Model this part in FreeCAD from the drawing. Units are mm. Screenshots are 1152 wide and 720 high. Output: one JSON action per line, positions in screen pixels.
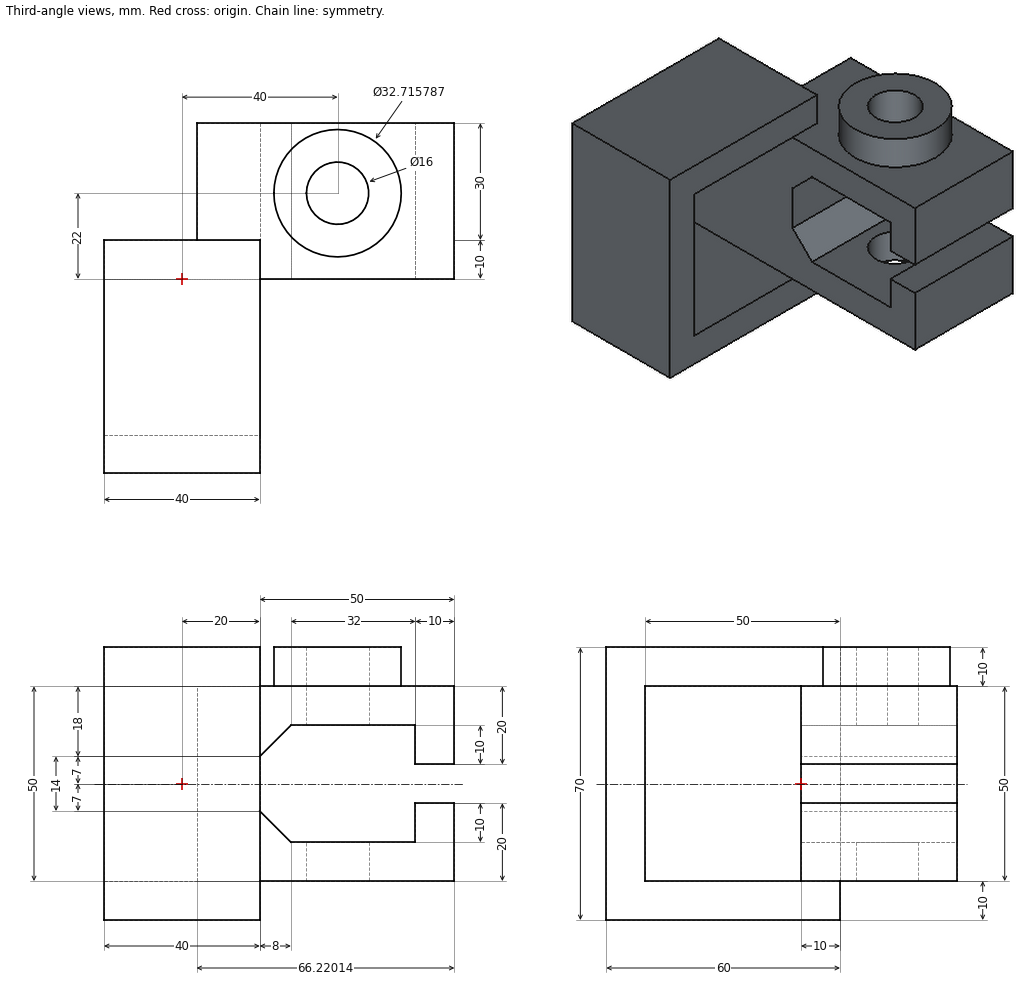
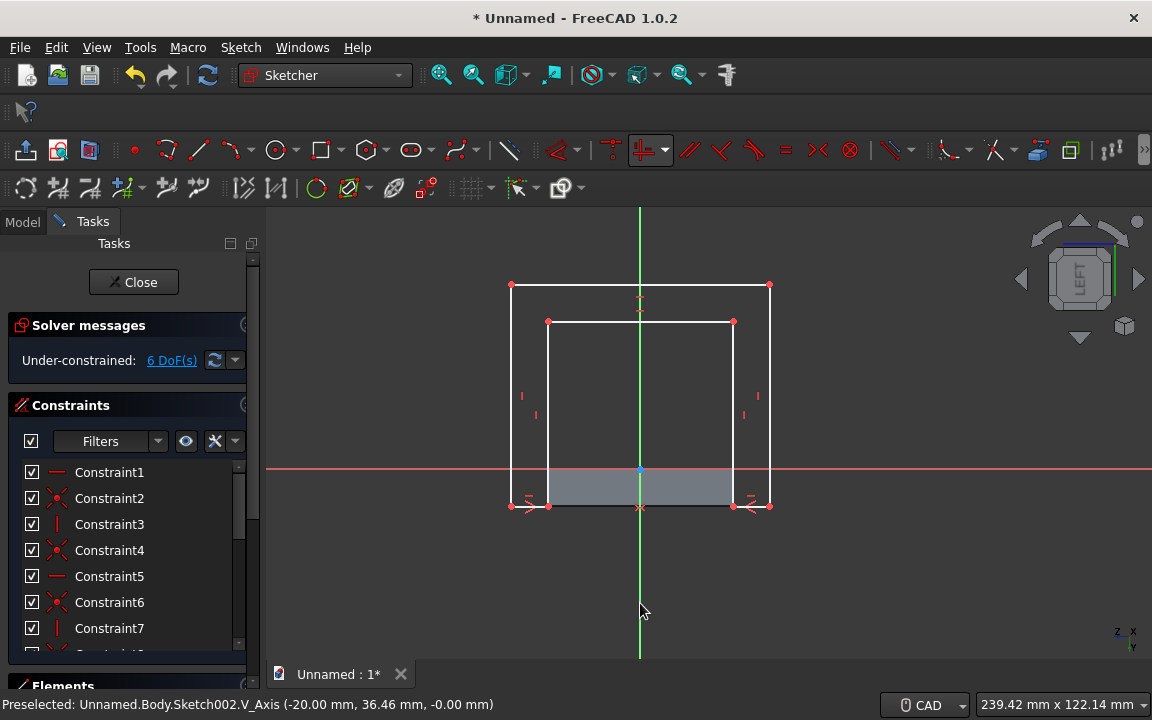
{"action": "key", "text": "d"}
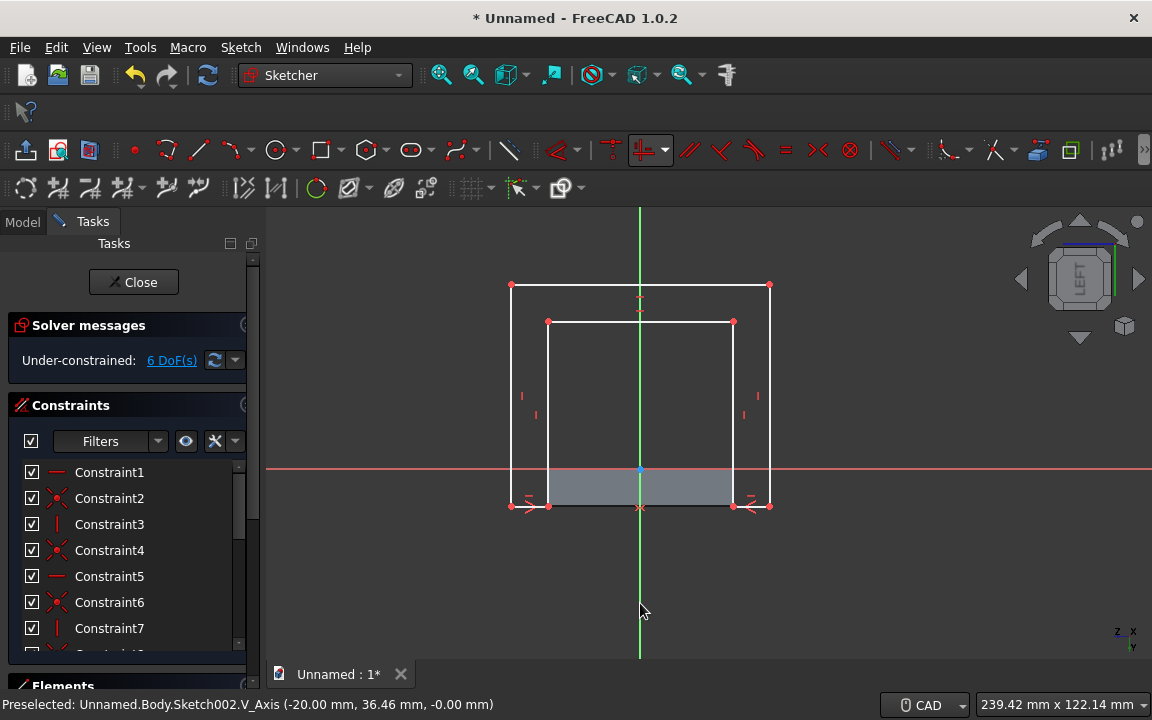
{"action": "scroll", "coordinate": [744, 507], "scroll_direction": "up", "scroll_amount": 2}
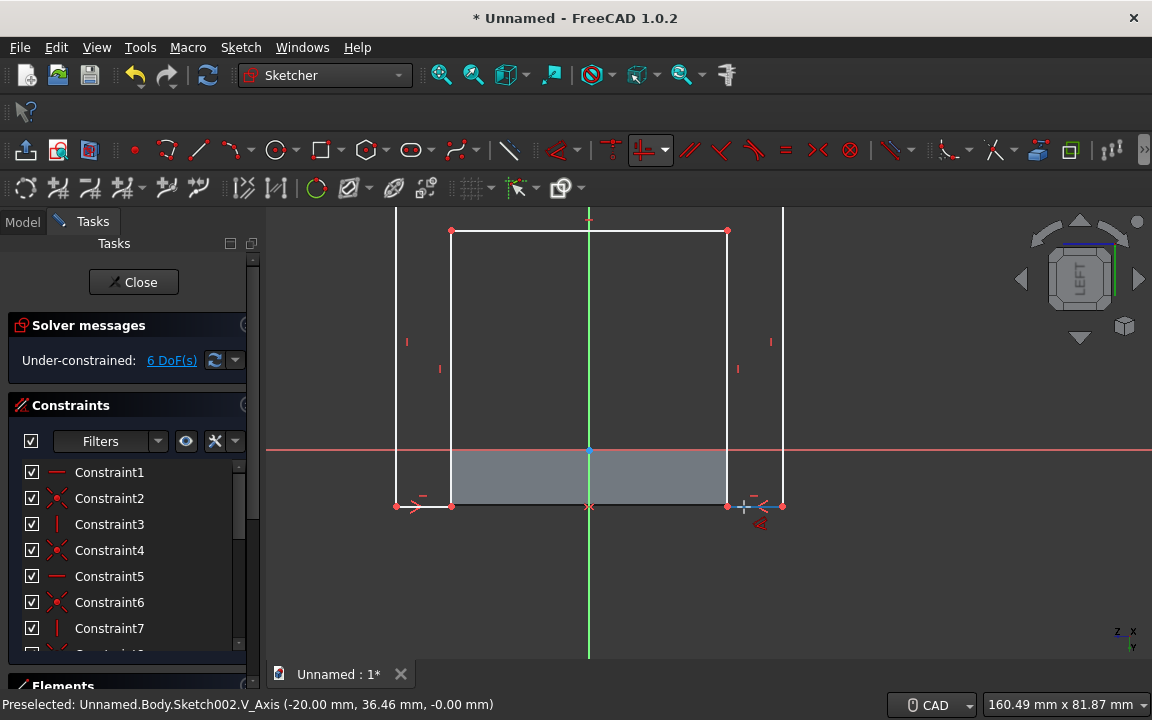
{"action": "left_click", "coordinate": [744, 507]}
{"action": "left_click", "coordinate": [755, 541]}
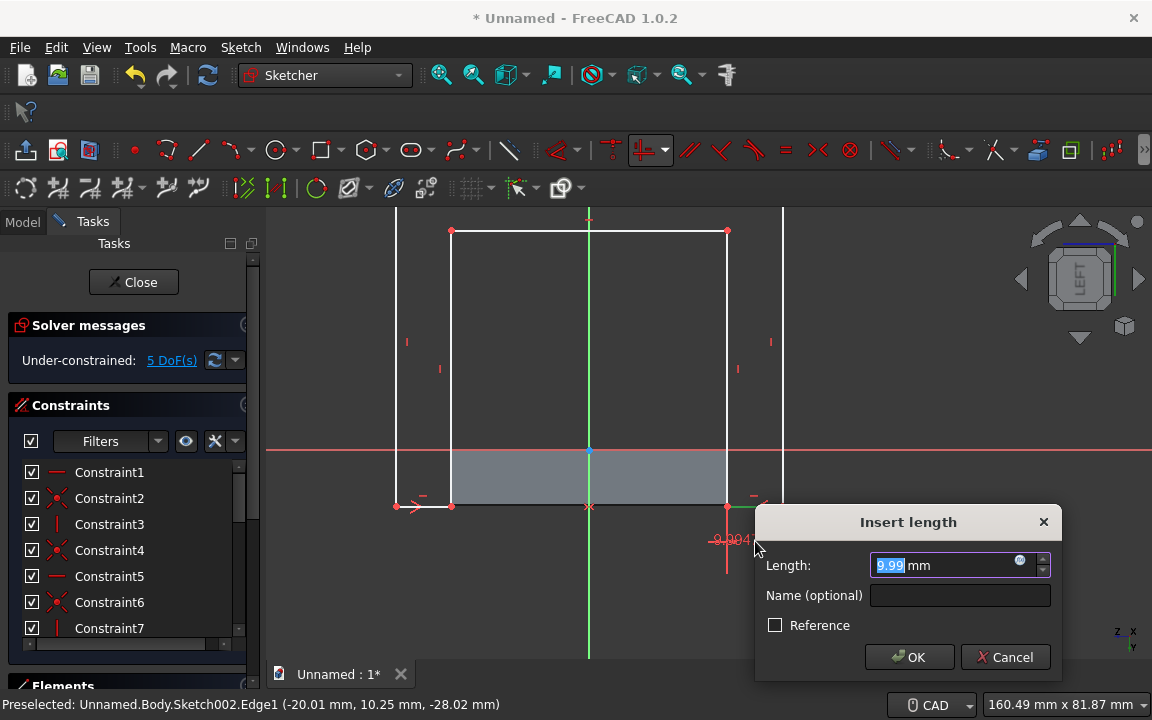
{"action": "type", "text": "10"}
{"action": "key", "text": "Return"}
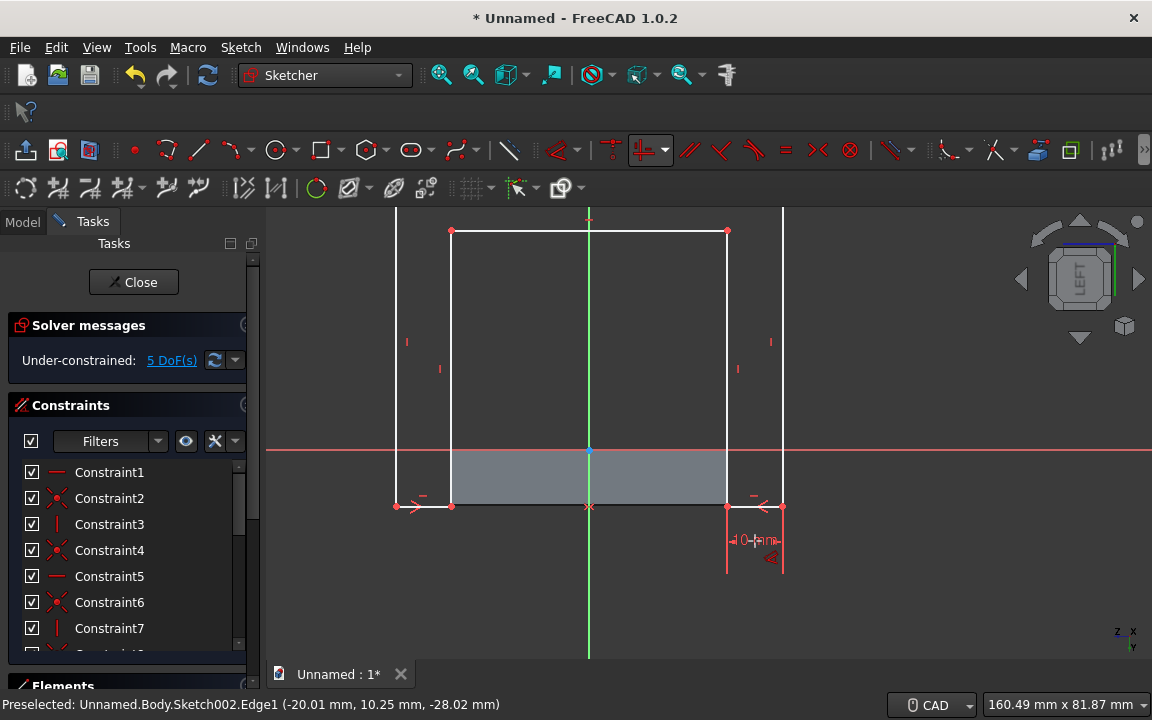
{"action": "left_click", "coordinate": [783, 407]}
{"action": "left_click", "coordinate": [817, 371]}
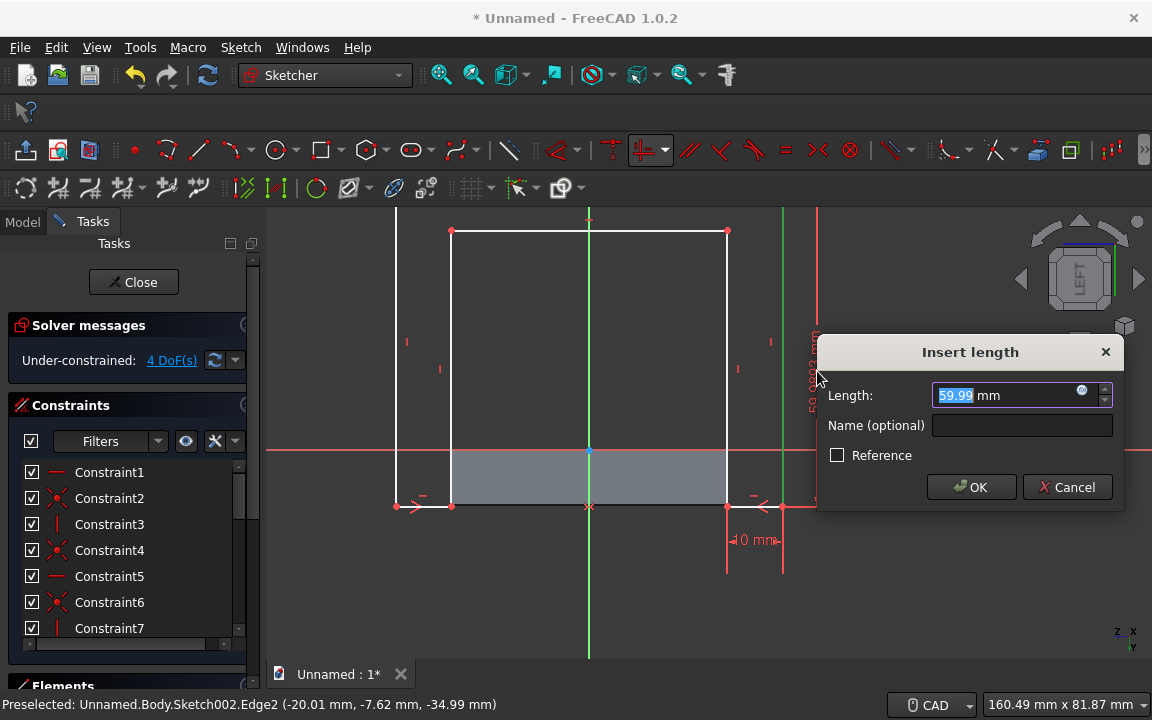
{"action": "type", "text": "60"}
{"action": "key", "text": "Return"}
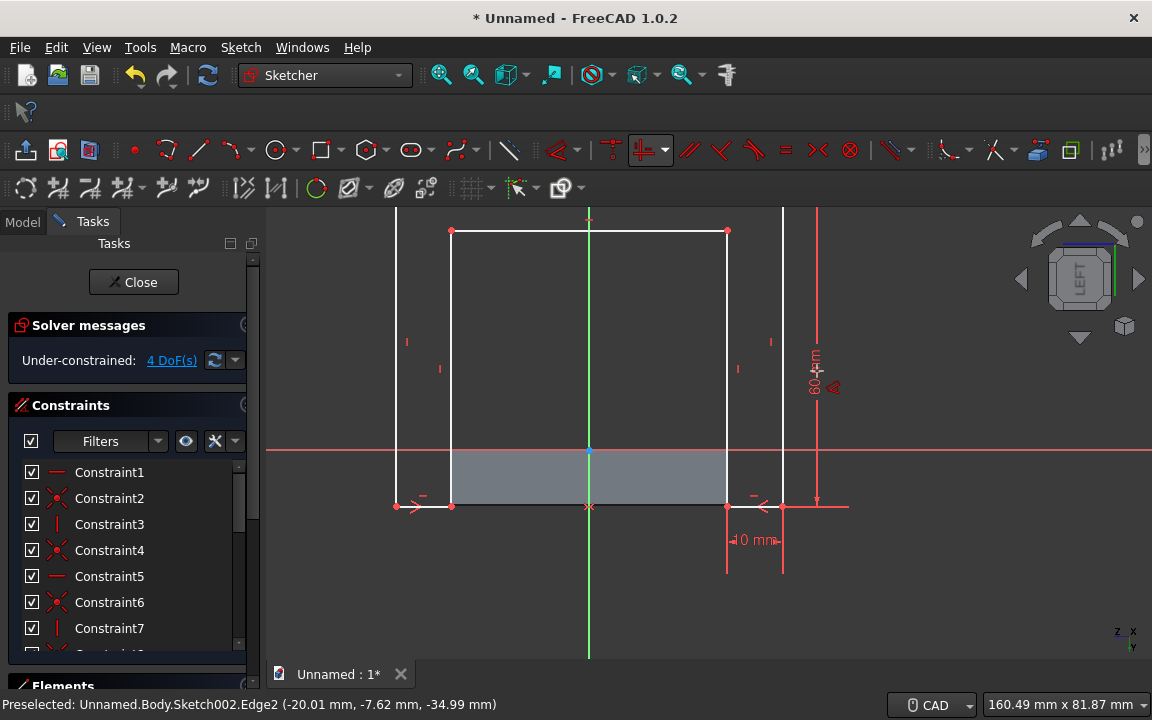
{"action": "scroll", "coordinate": [745, 623], "scroll_direction": "down", "scroll_amount": 2}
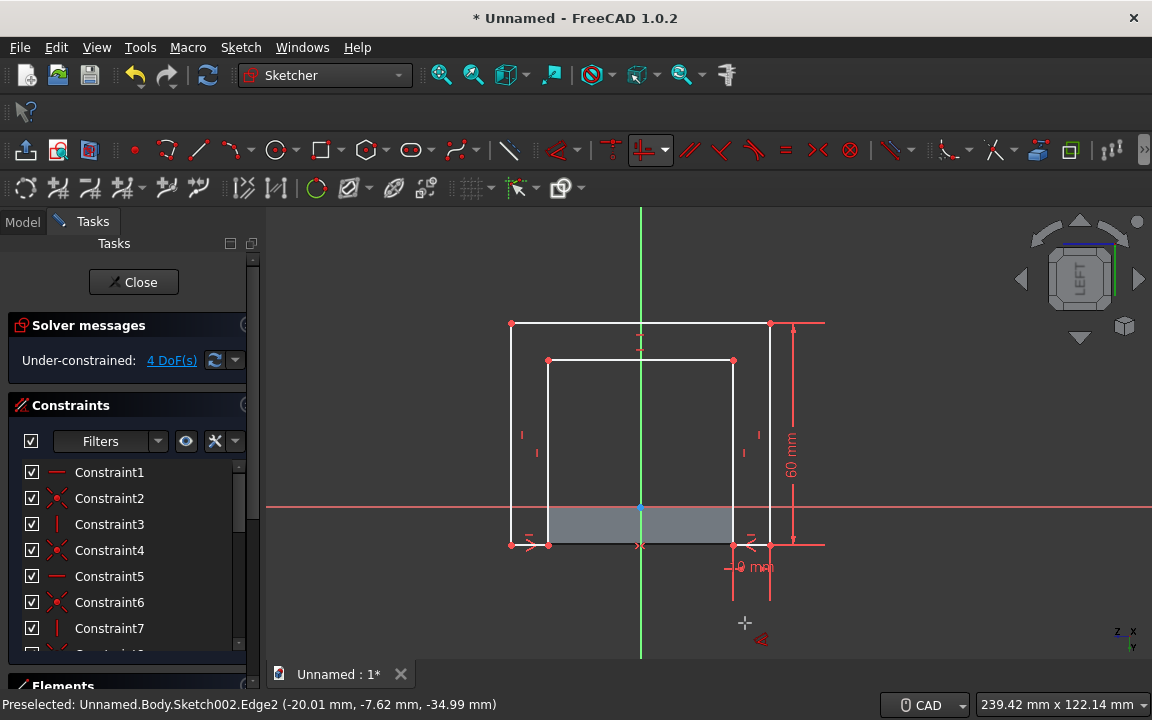
{"action": "left_click", "coordinate": [693, 323]}
{"action": "left_click", "coordinate": [581, 289]}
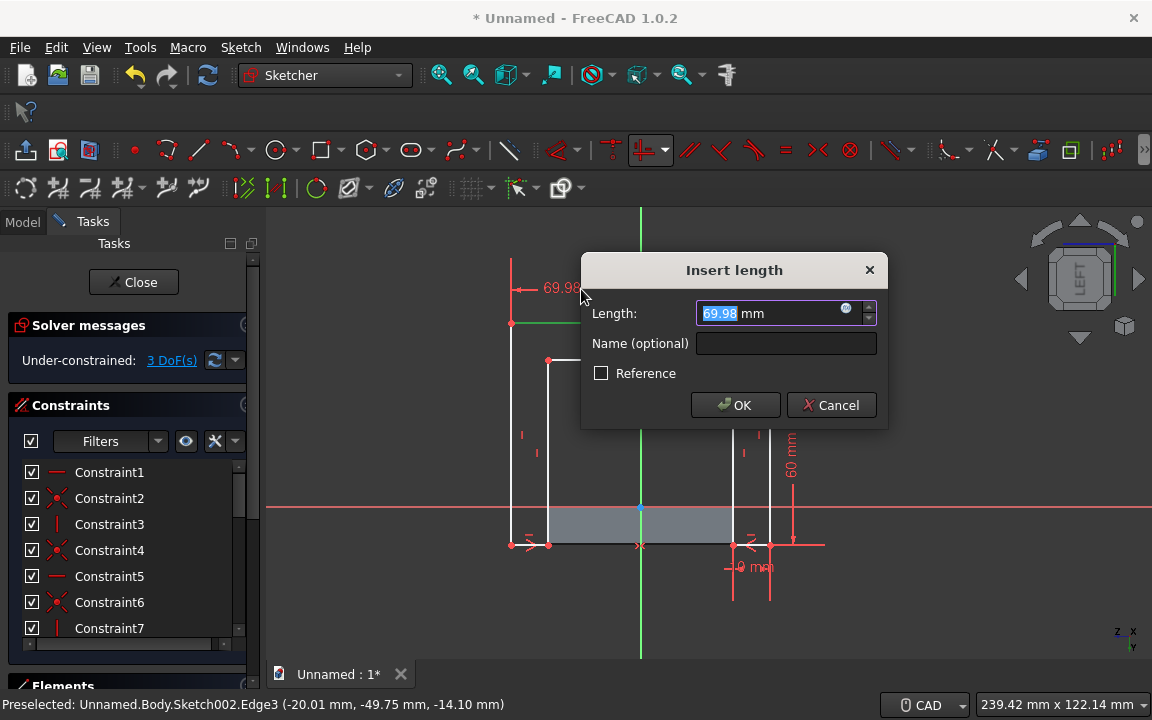
{"action": "type", "text": "70"}
{"action": "key", "text": "Return"}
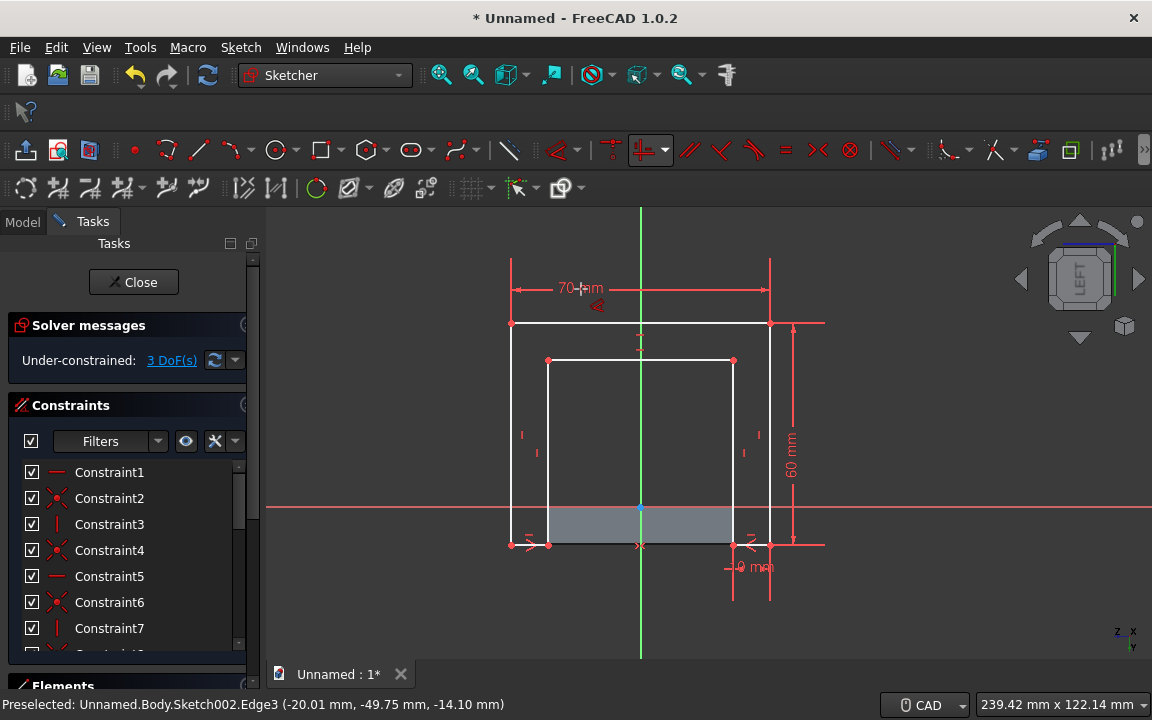
{"action": "scroll", "coordinate": [522, 545], "scroll_direction": "up", "scroll_amount": 2}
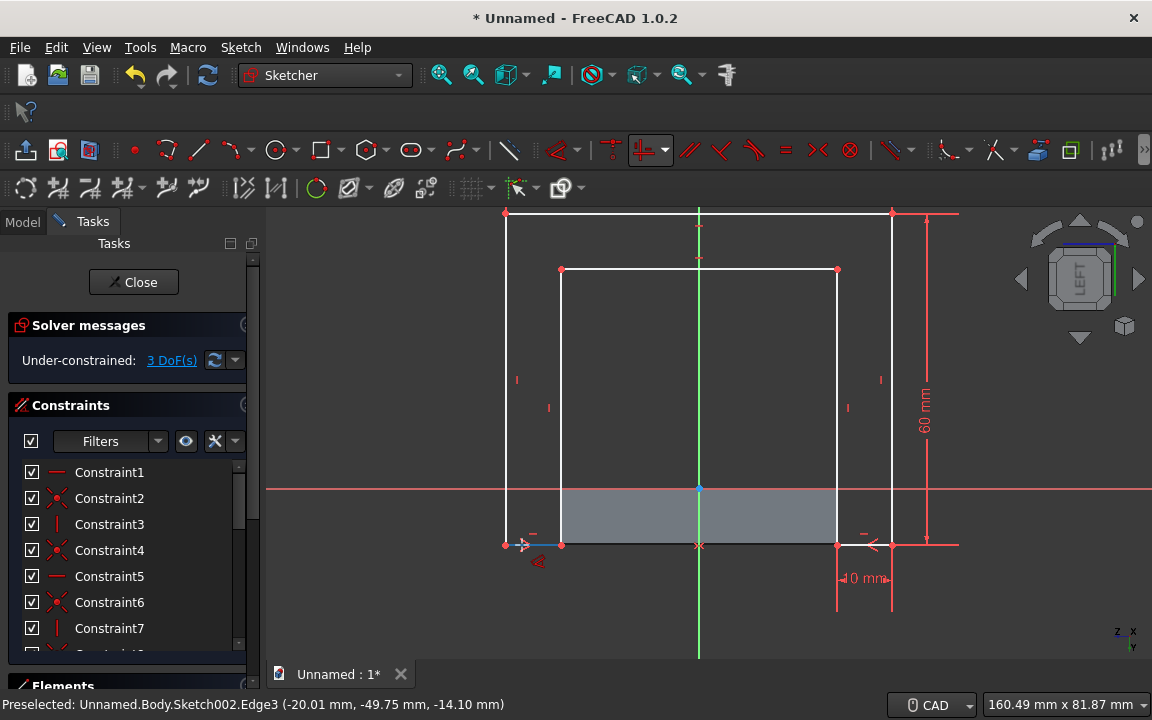
{"action": "left_click", "coordinate": [522, 545]}
{"action": "left_click", "coordinate": [534, 579]}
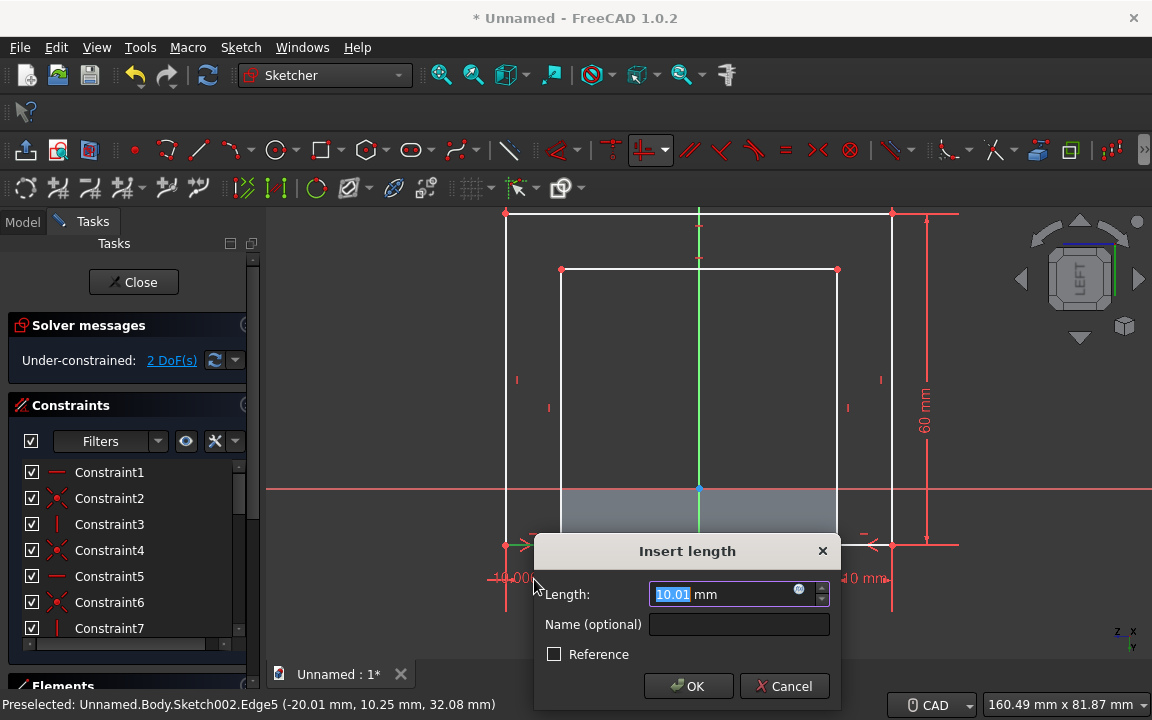
{"action": "type", "text": "10"}
{"action": "key", "text": "Return"}